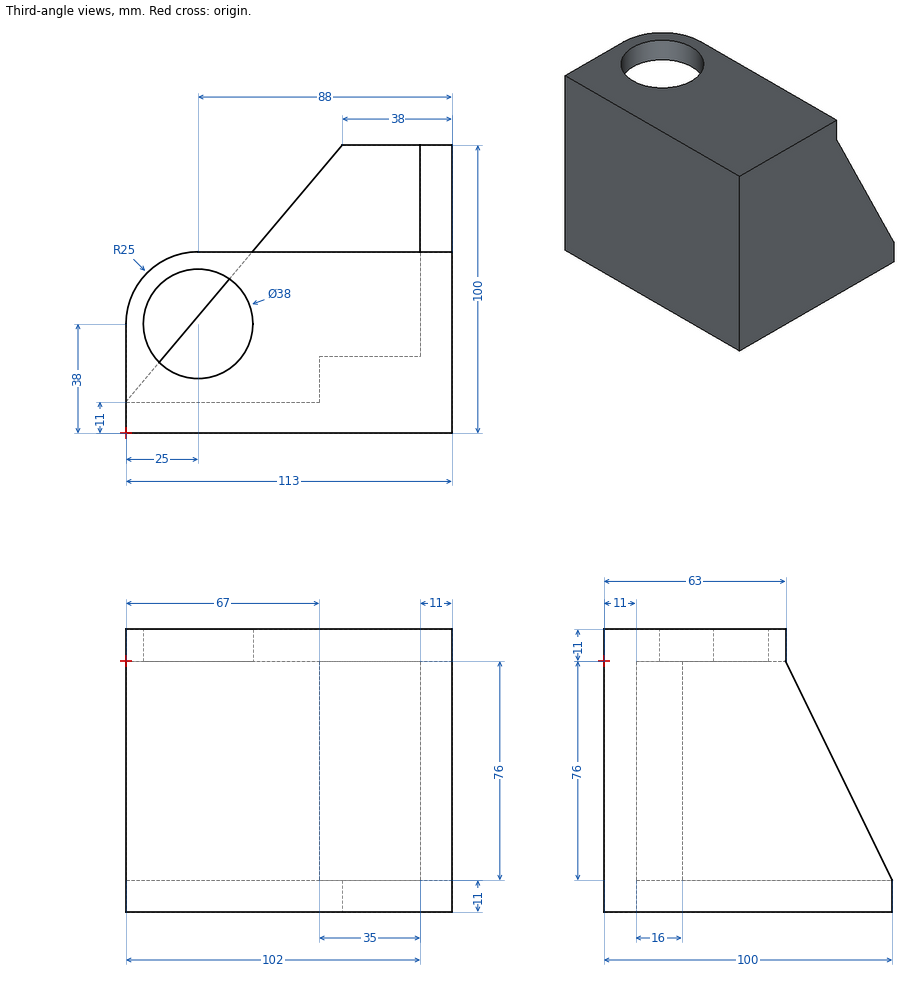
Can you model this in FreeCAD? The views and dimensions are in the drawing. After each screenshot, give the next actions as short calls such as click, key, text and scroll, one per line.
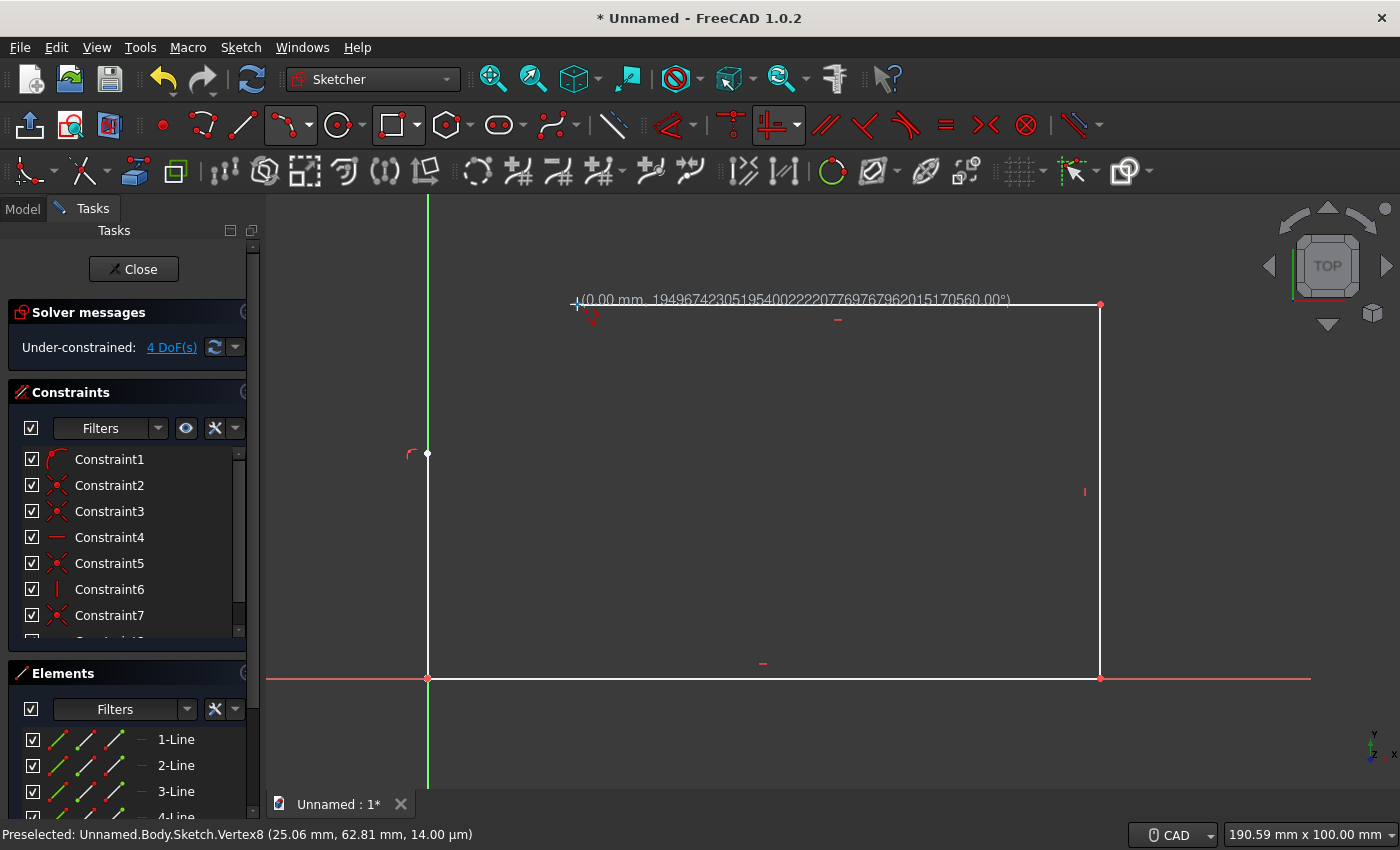
click(284, 126)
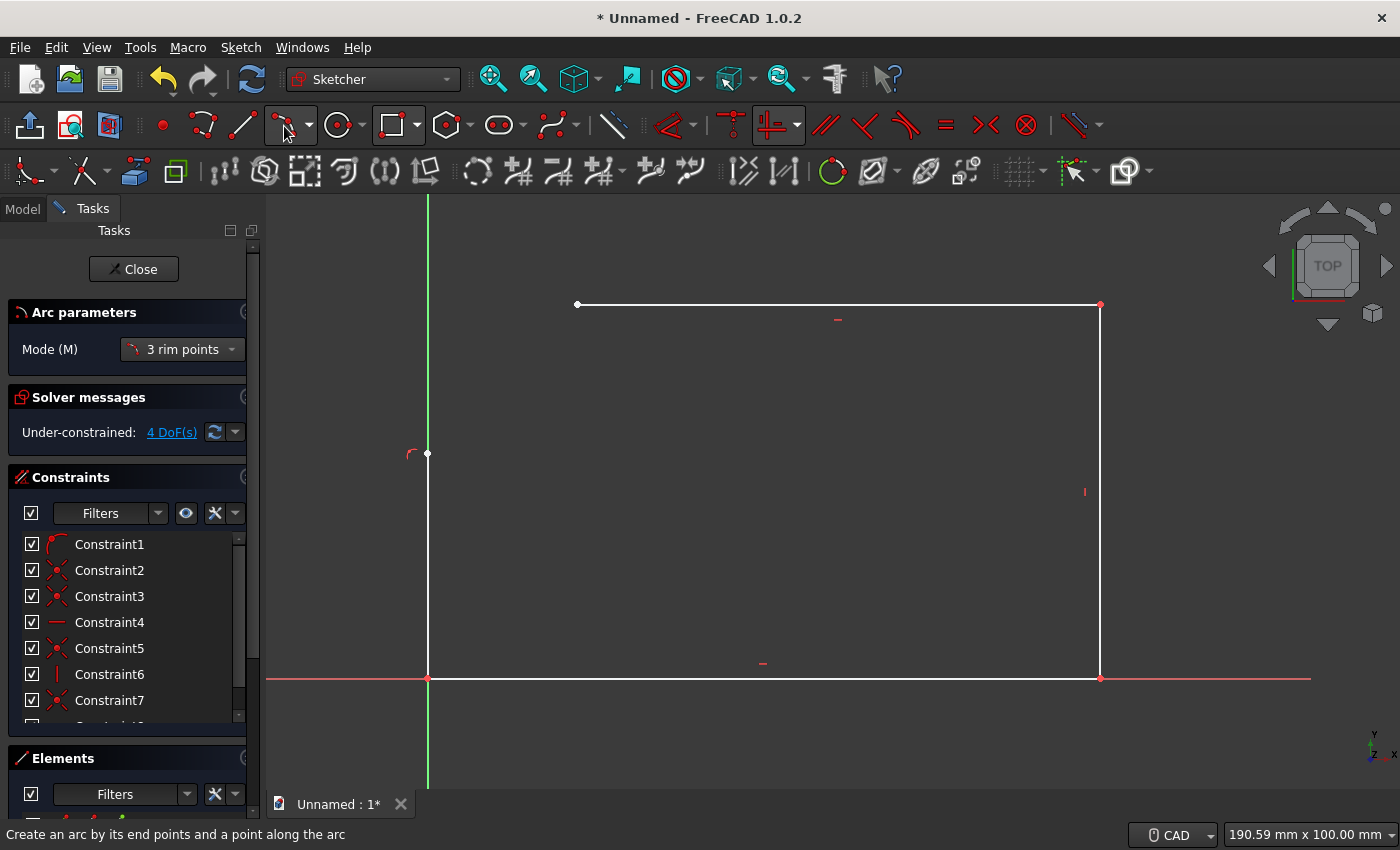
click(577, 305)
click(428, 454)
click(471, 347)
key(Escape)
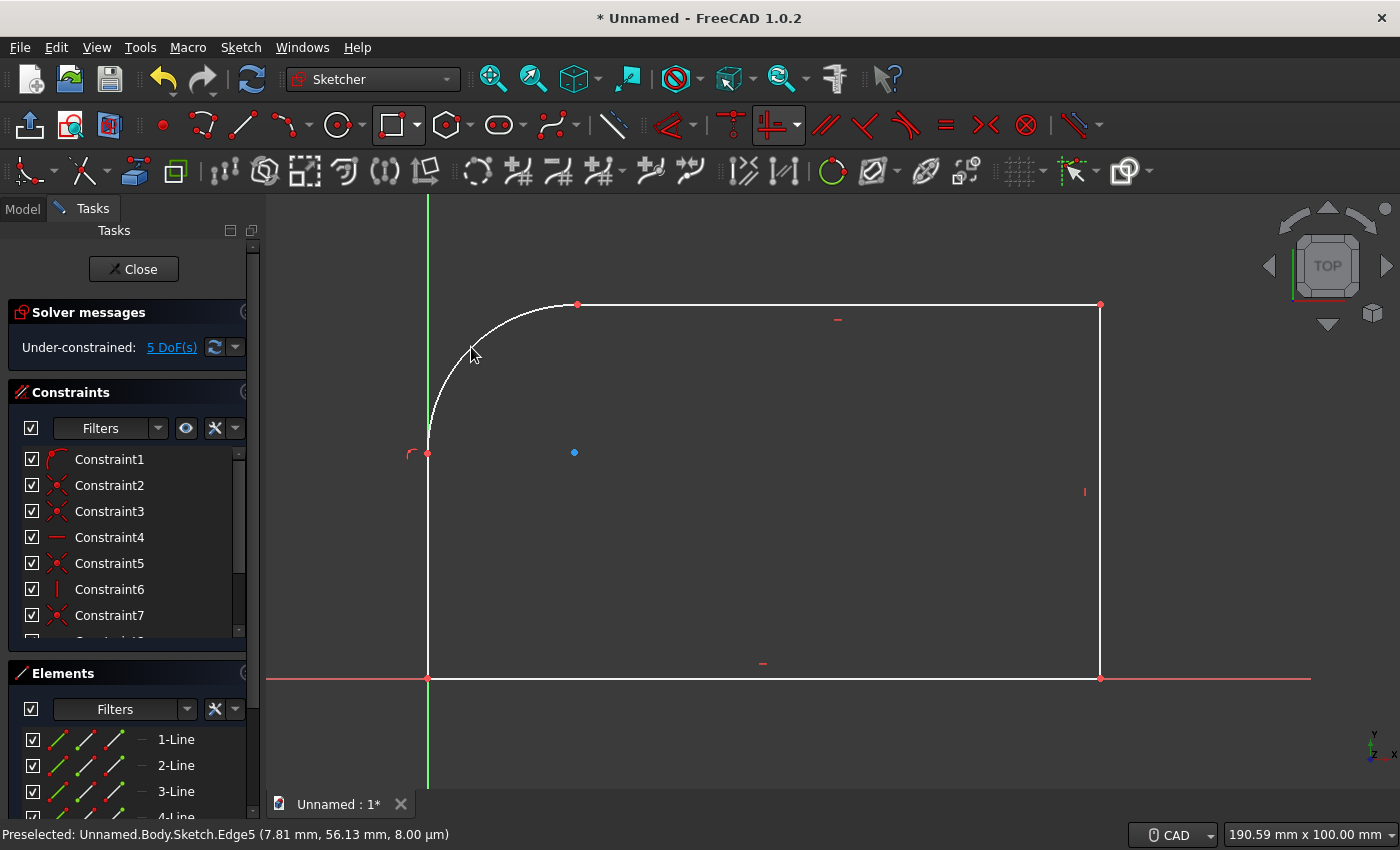
click(428, 521)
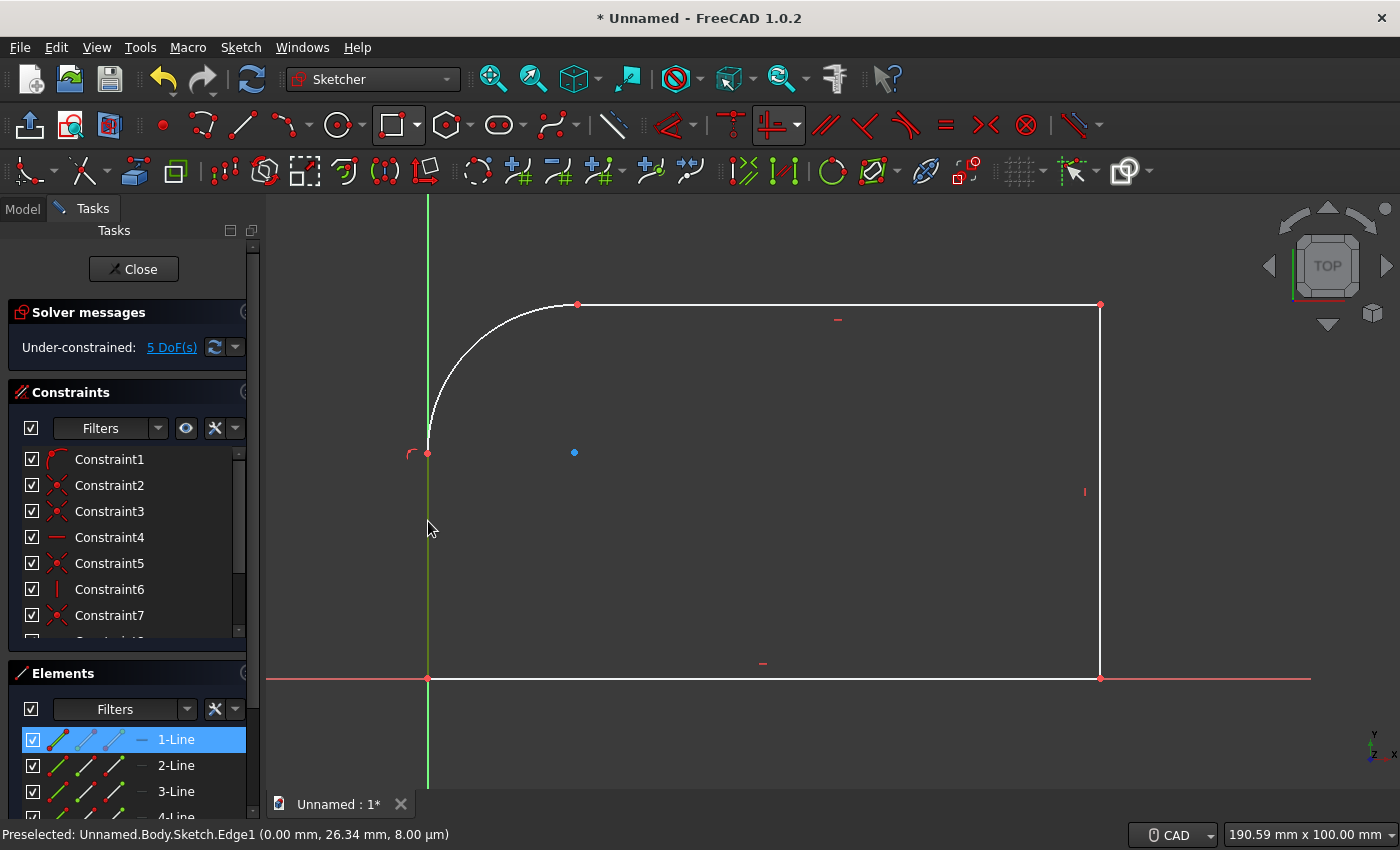
click(509, 321)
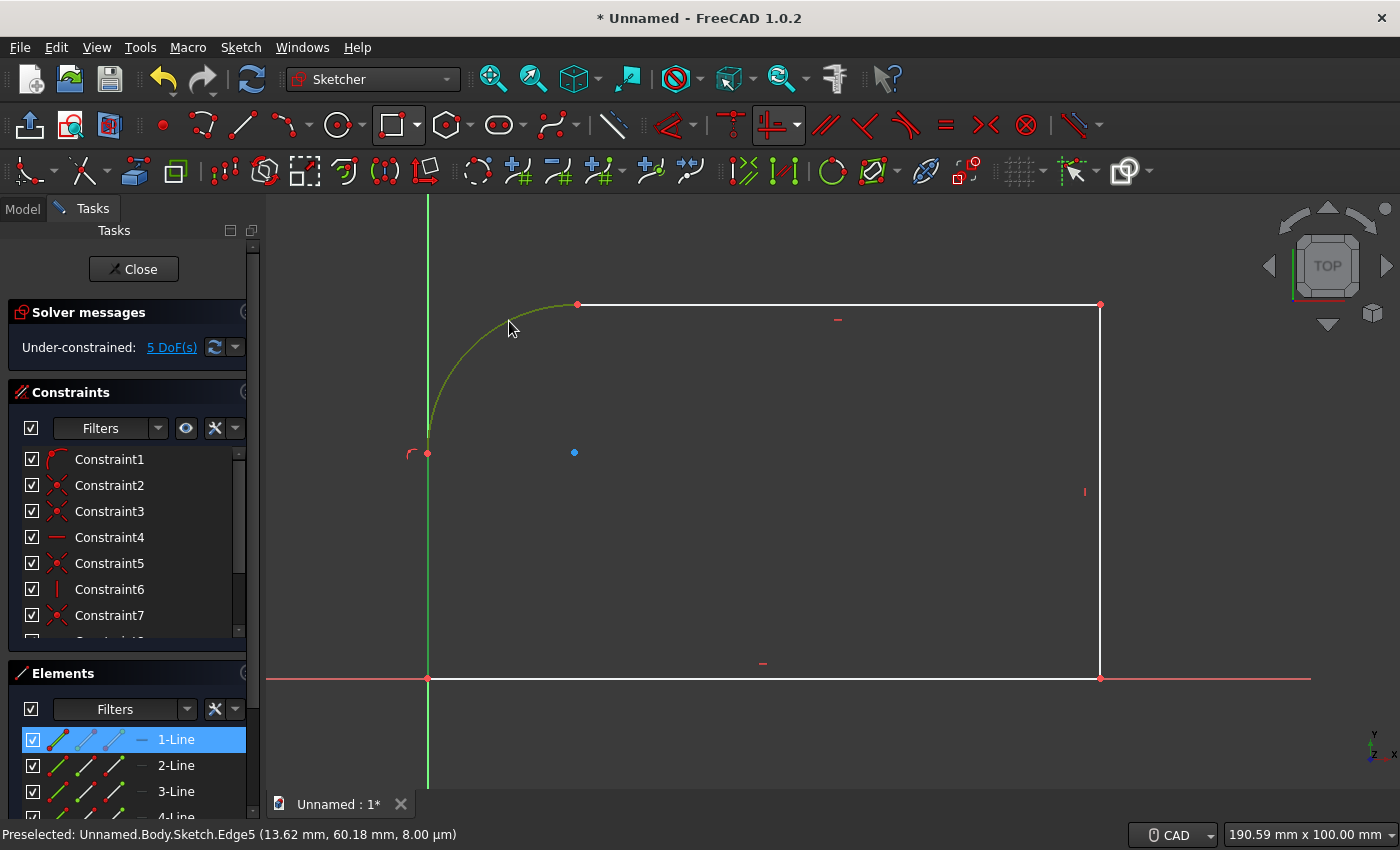
click(906, 126)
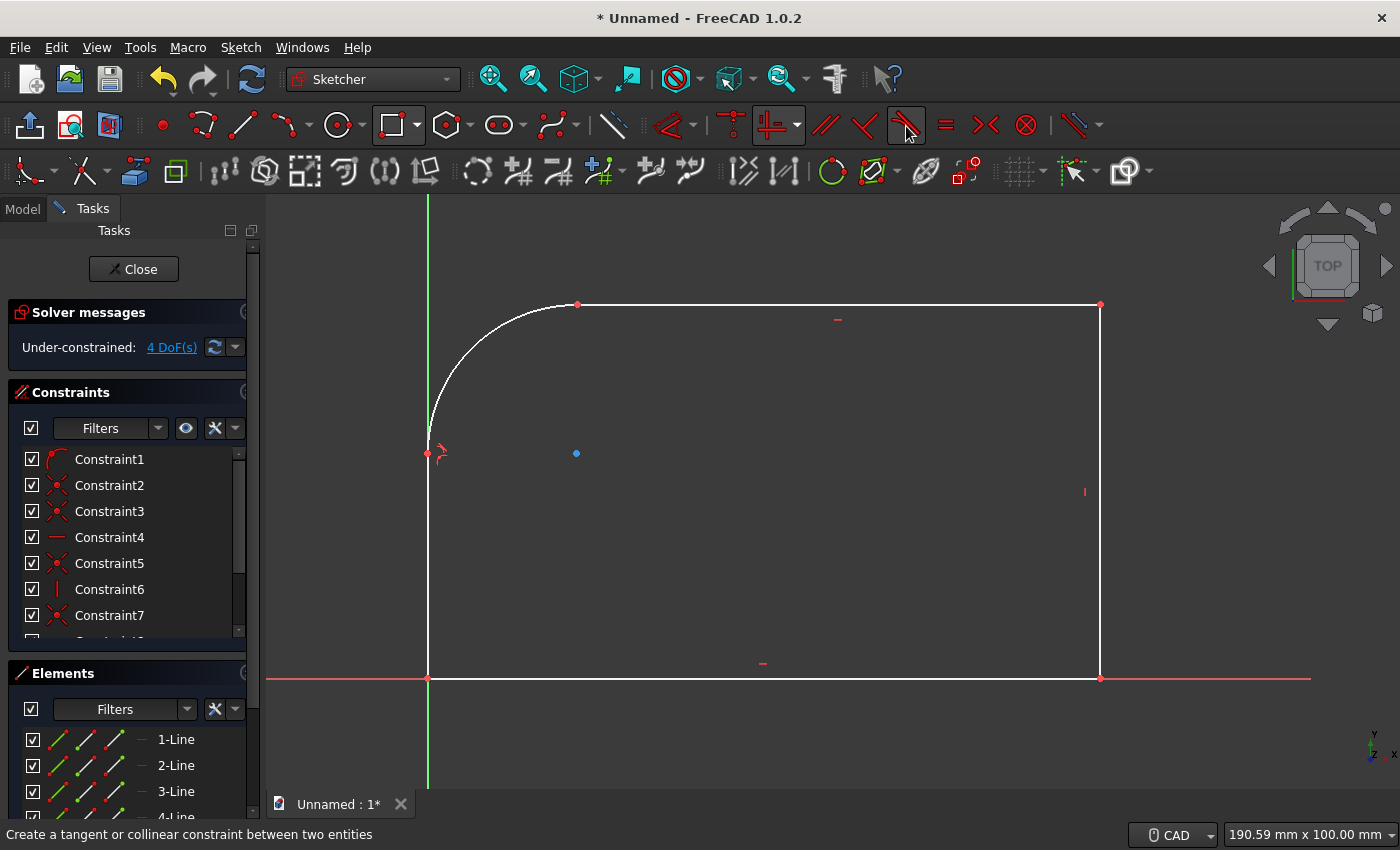
click(943, 305)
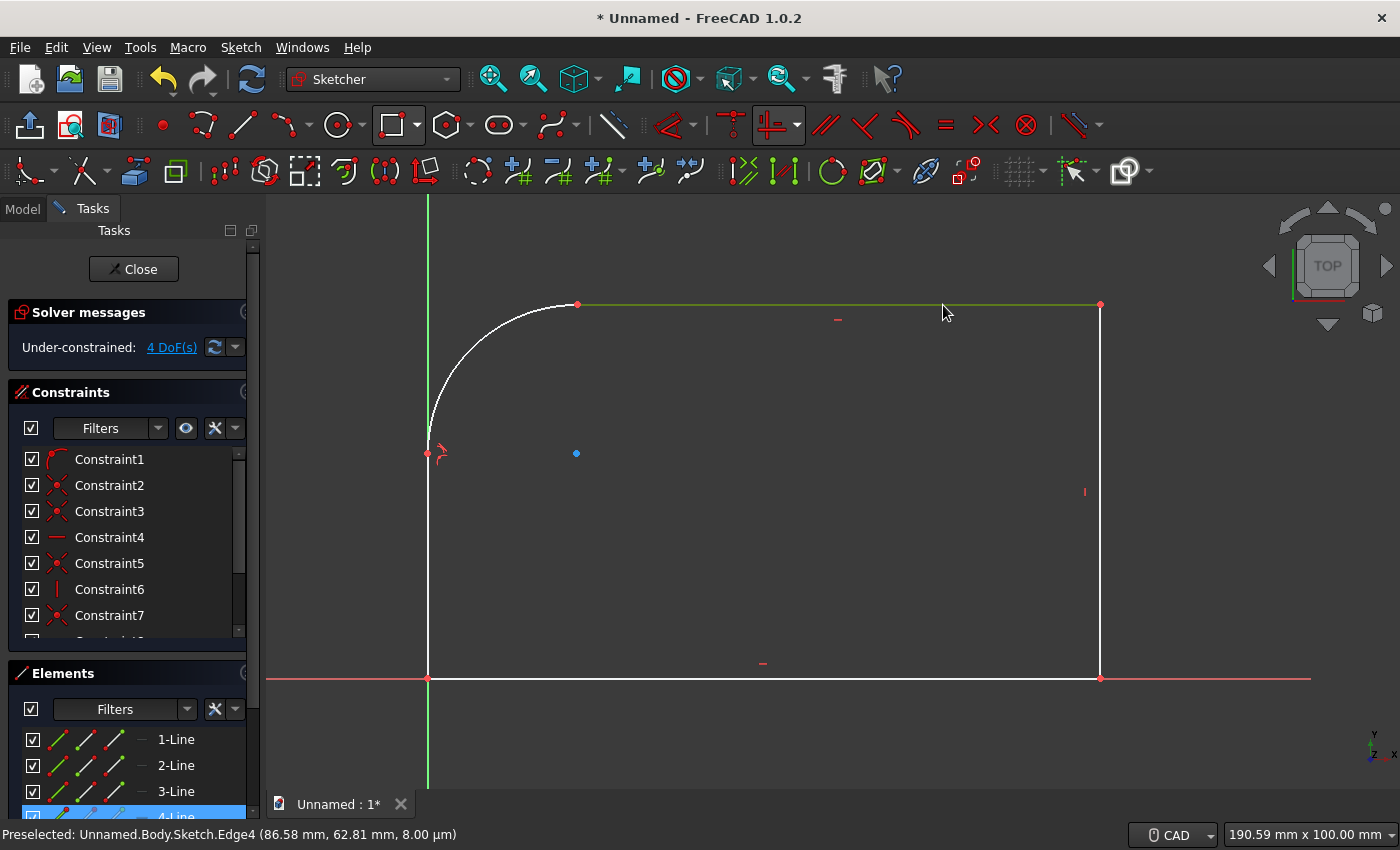
click(509, 321)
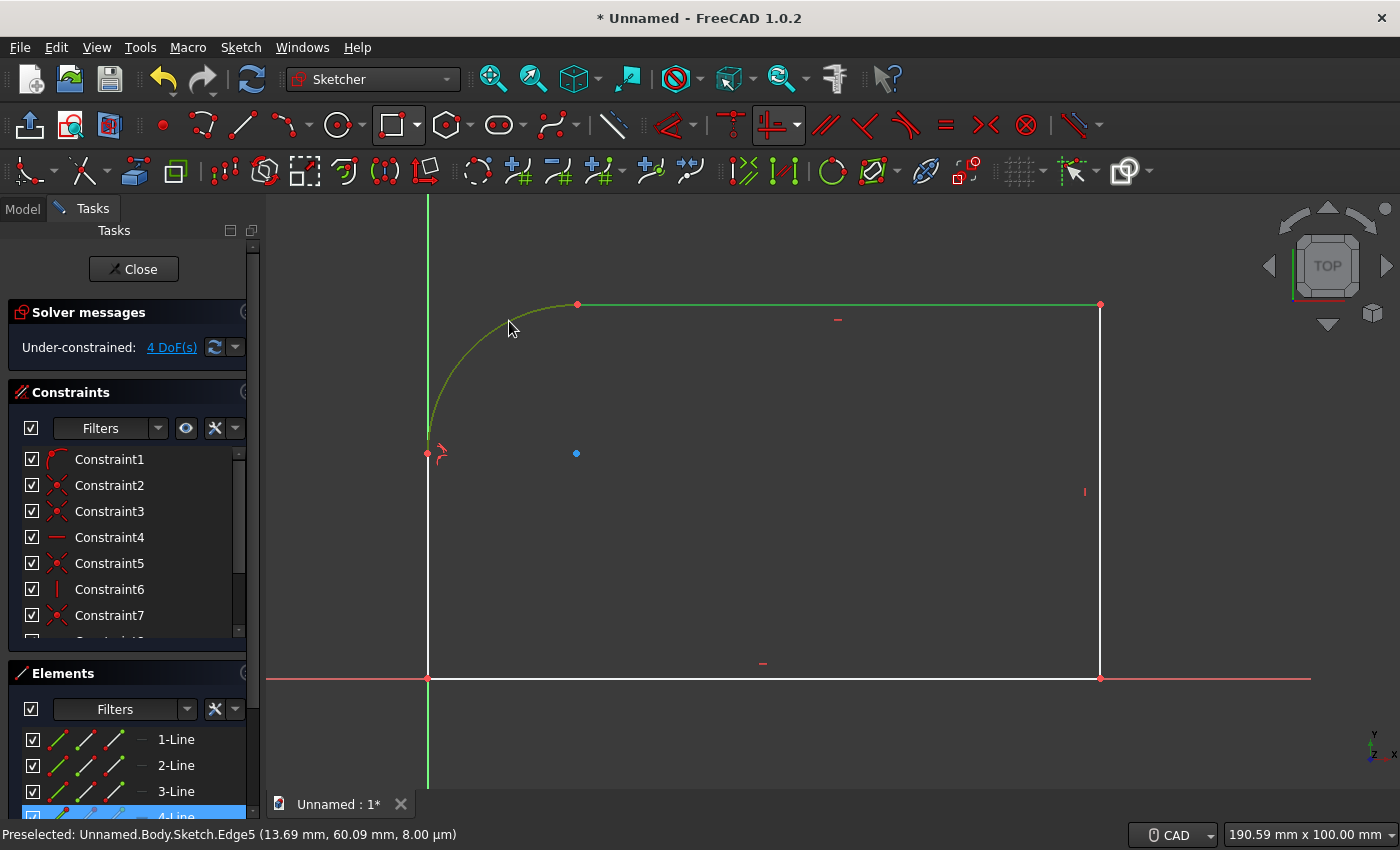
key(t)